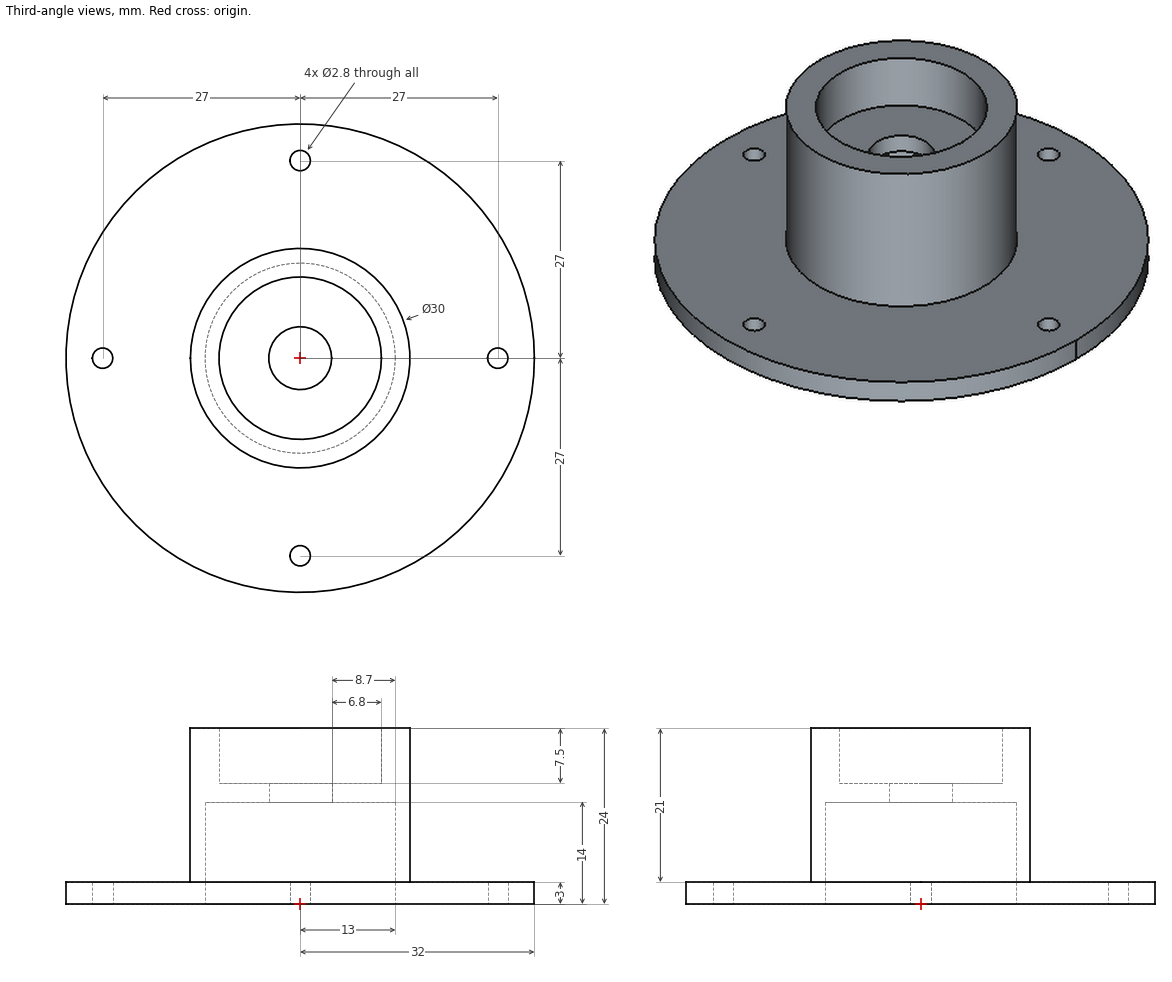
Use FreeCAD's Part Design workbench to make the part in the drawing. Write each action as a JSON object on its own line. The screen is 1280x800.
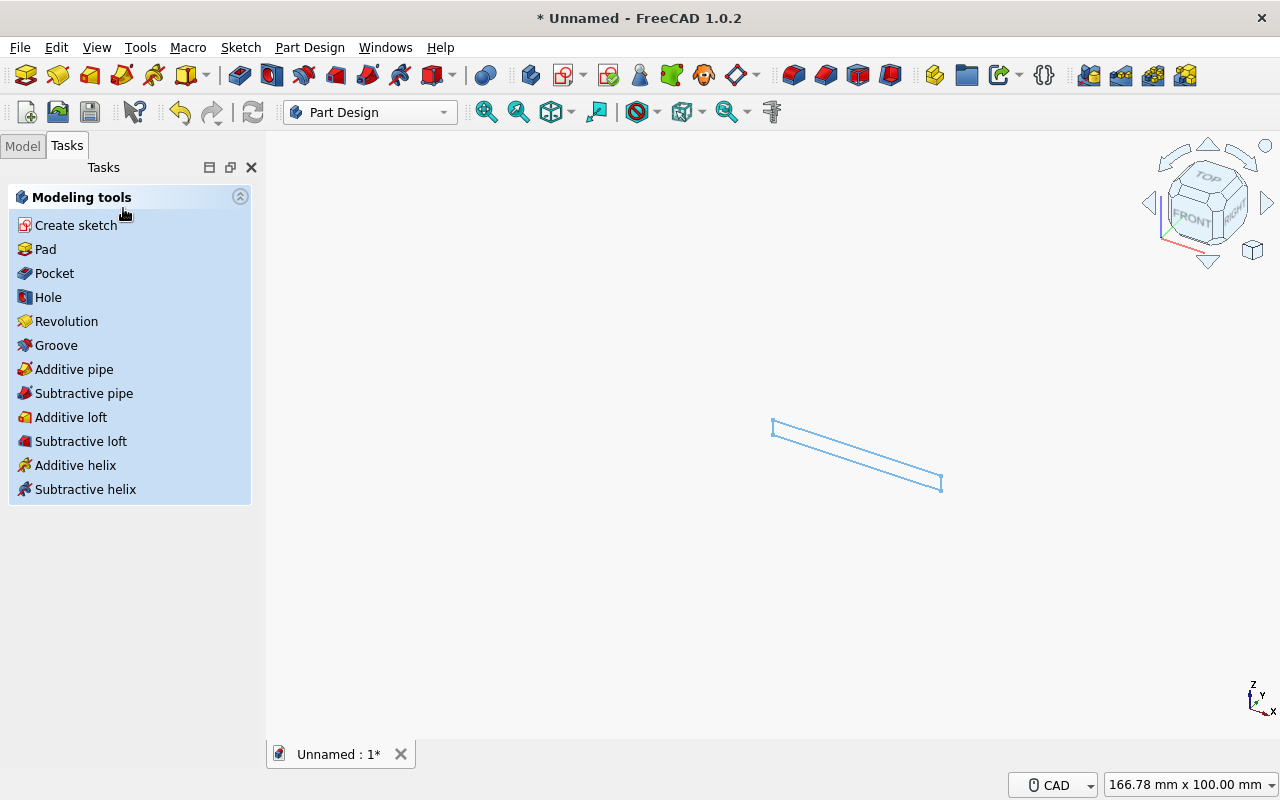
{"action": "left_click", "coordinate": [58, 76]}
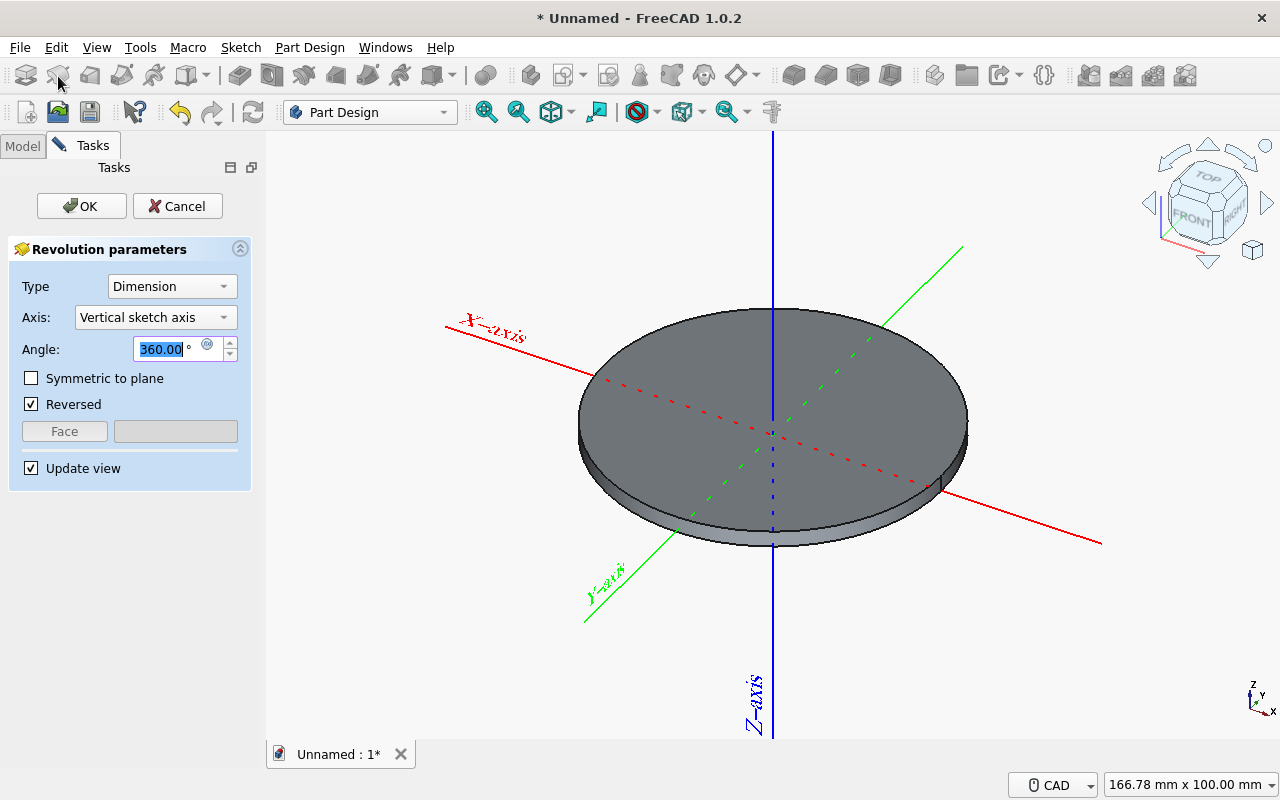
{"action": "left_click", "coordinate": [82, 206]}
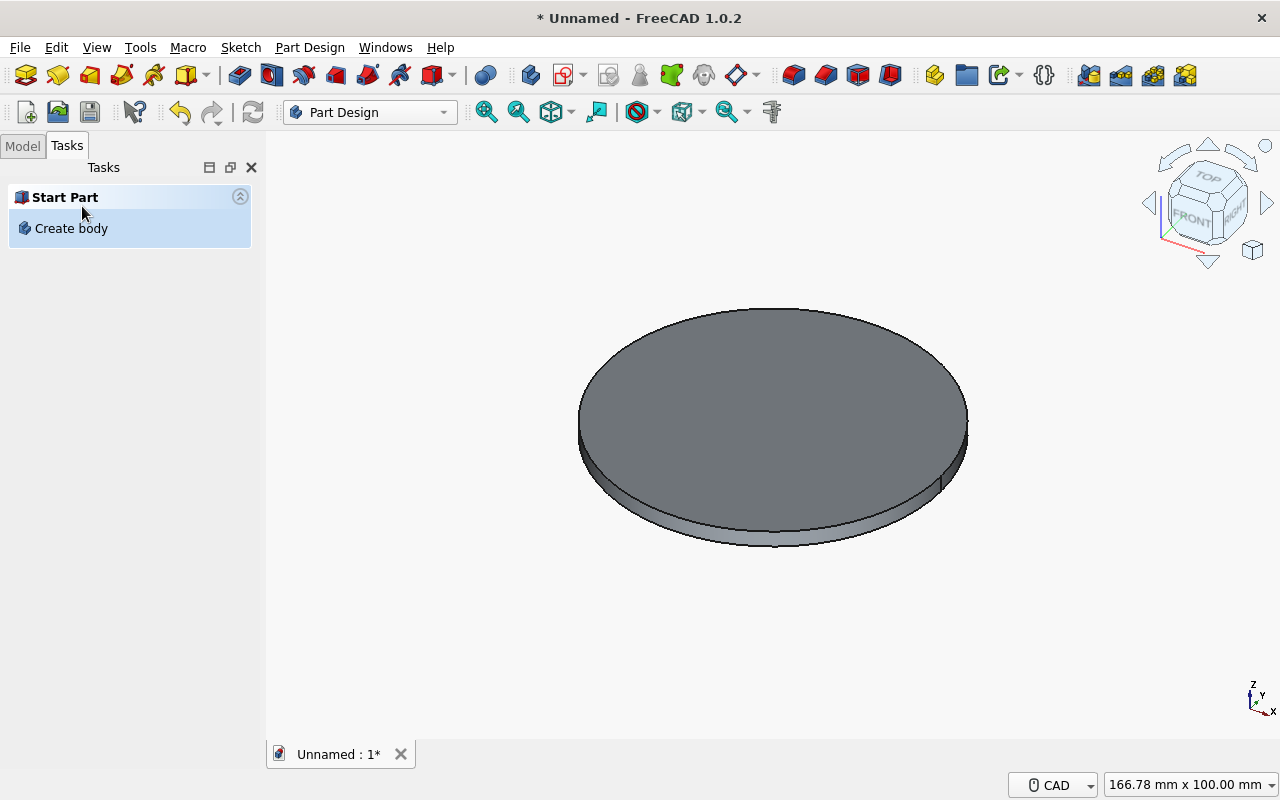
{"action": "left_click", "coordinate": [773, 419]}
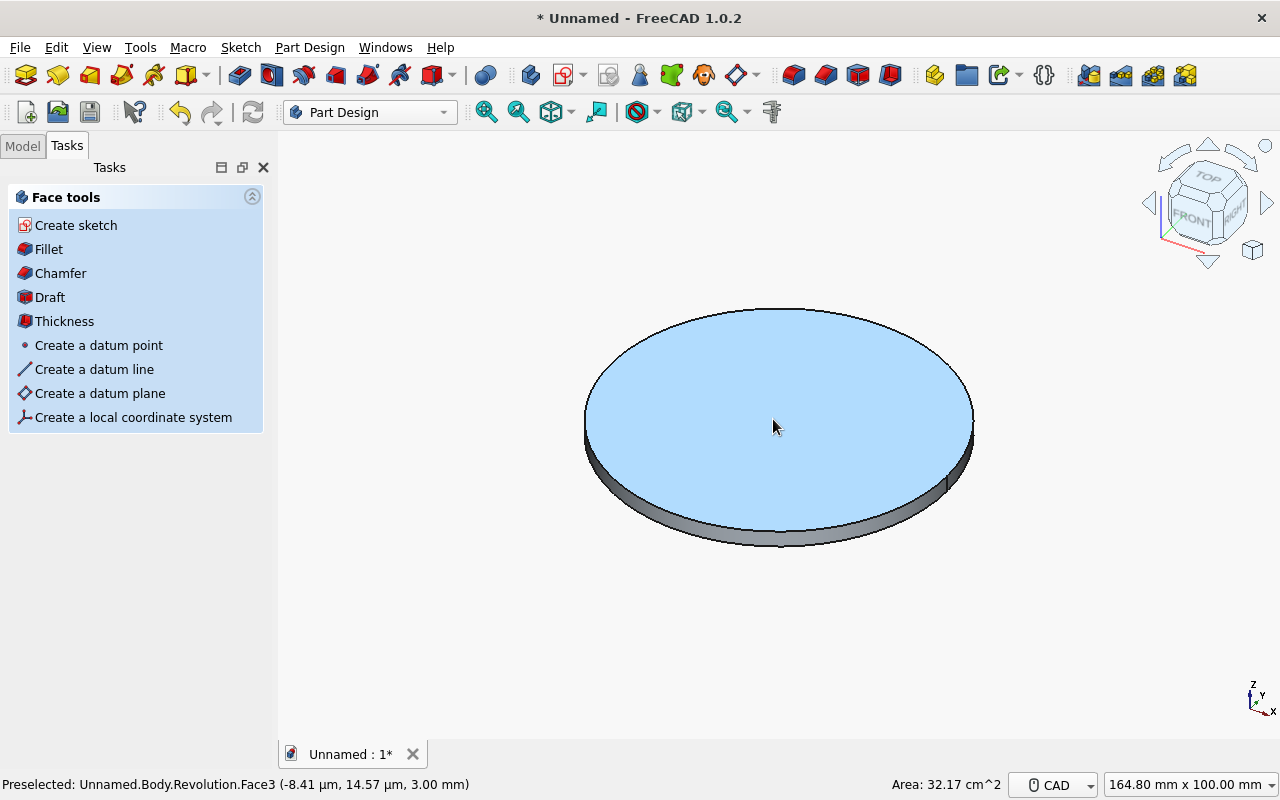
{"action": "left_click", "coordinate": [564, 76]}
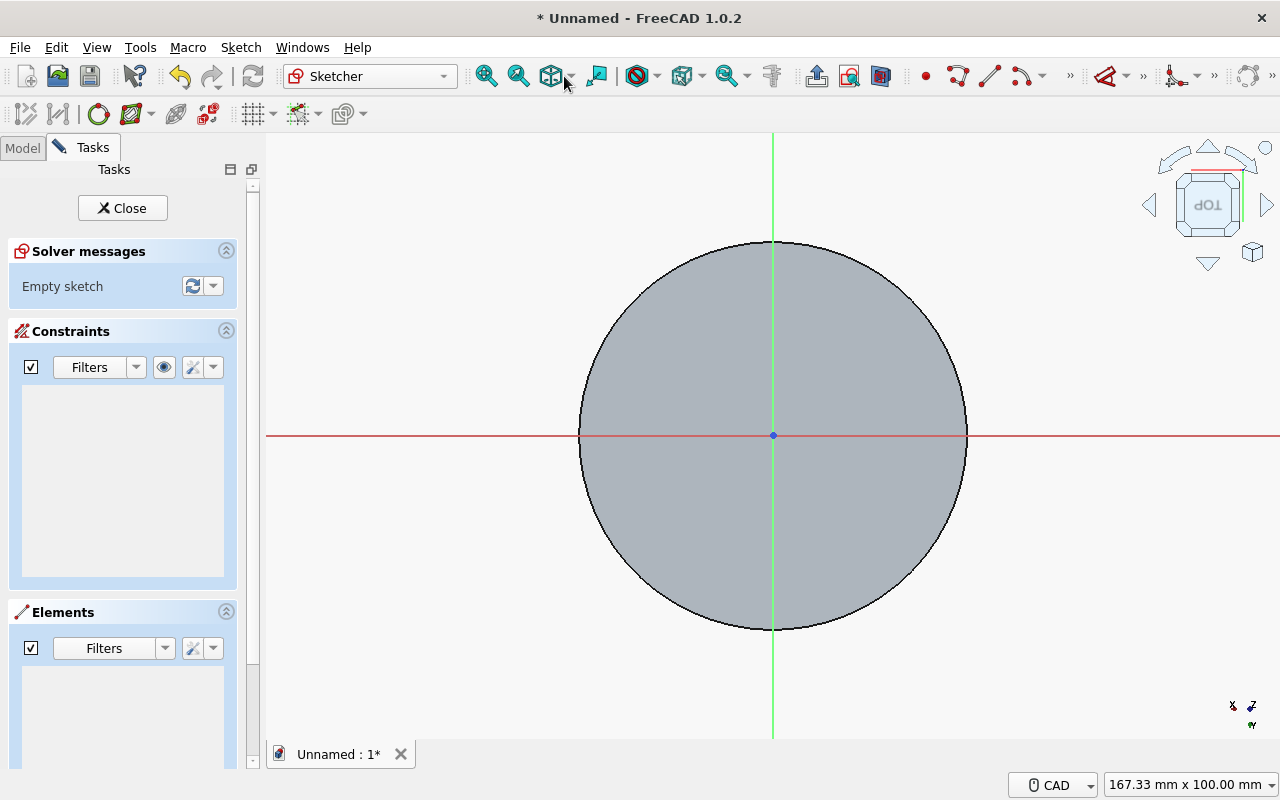
{"action": "scroll", "coordinate": [829, 436], "scroll_direction": "up", "scroll_amount": 4}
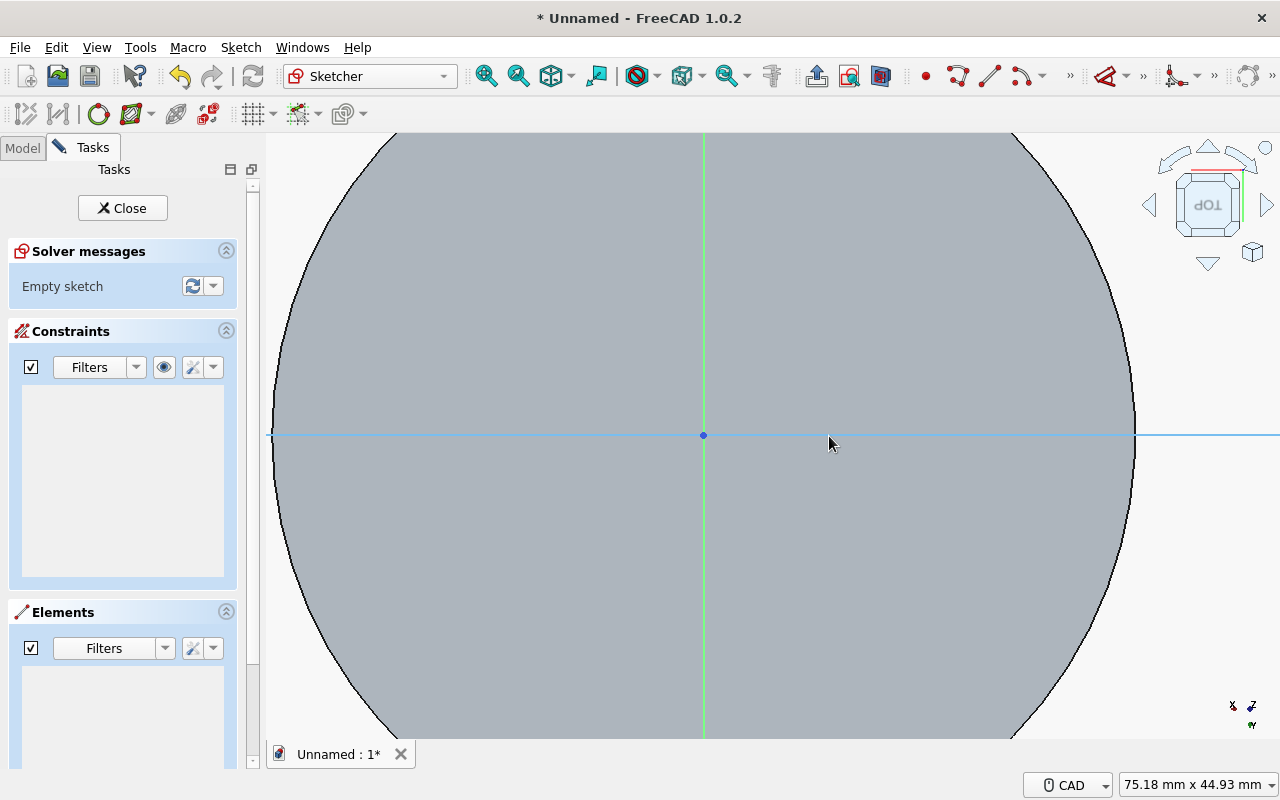
{"action": "key", "text": "g c"}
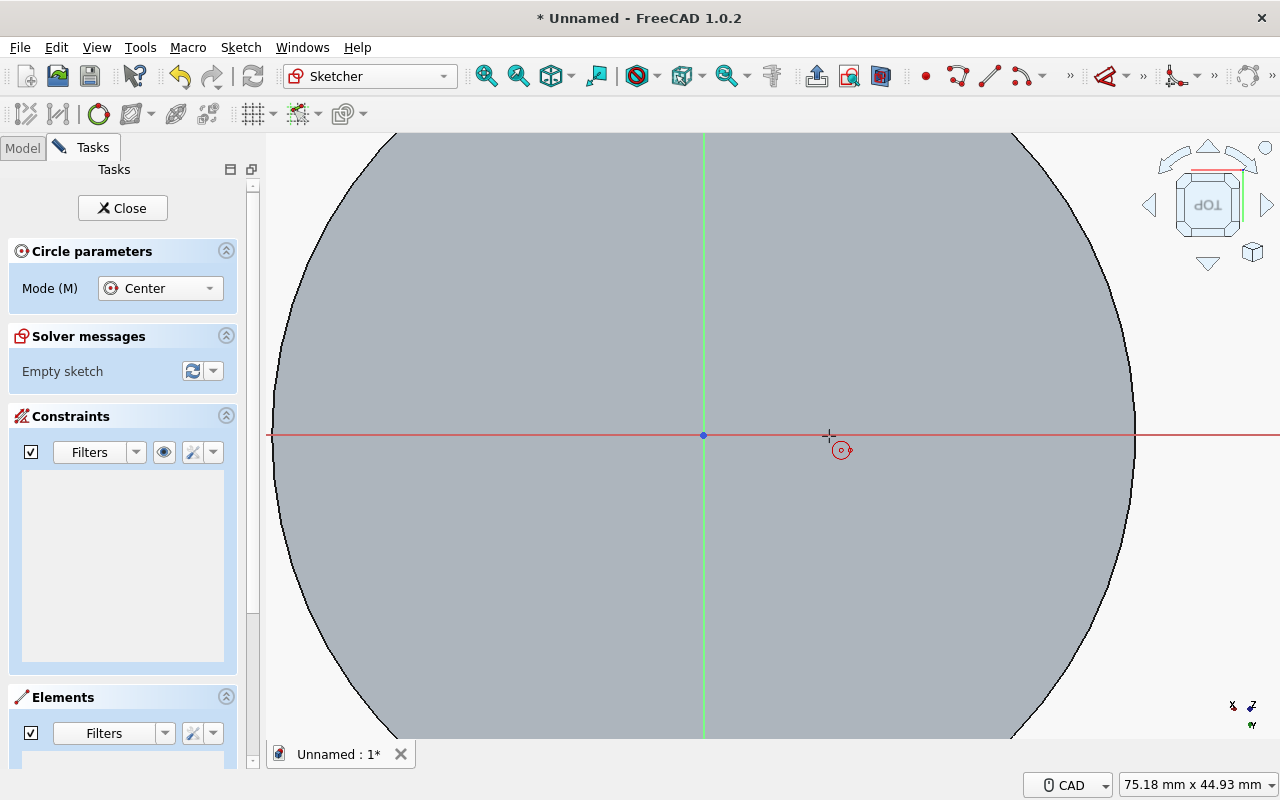
{"action": "left_click", "coordinate": [704, 435]}
{"action": "mouse_move", "coordinate": [847, 292]}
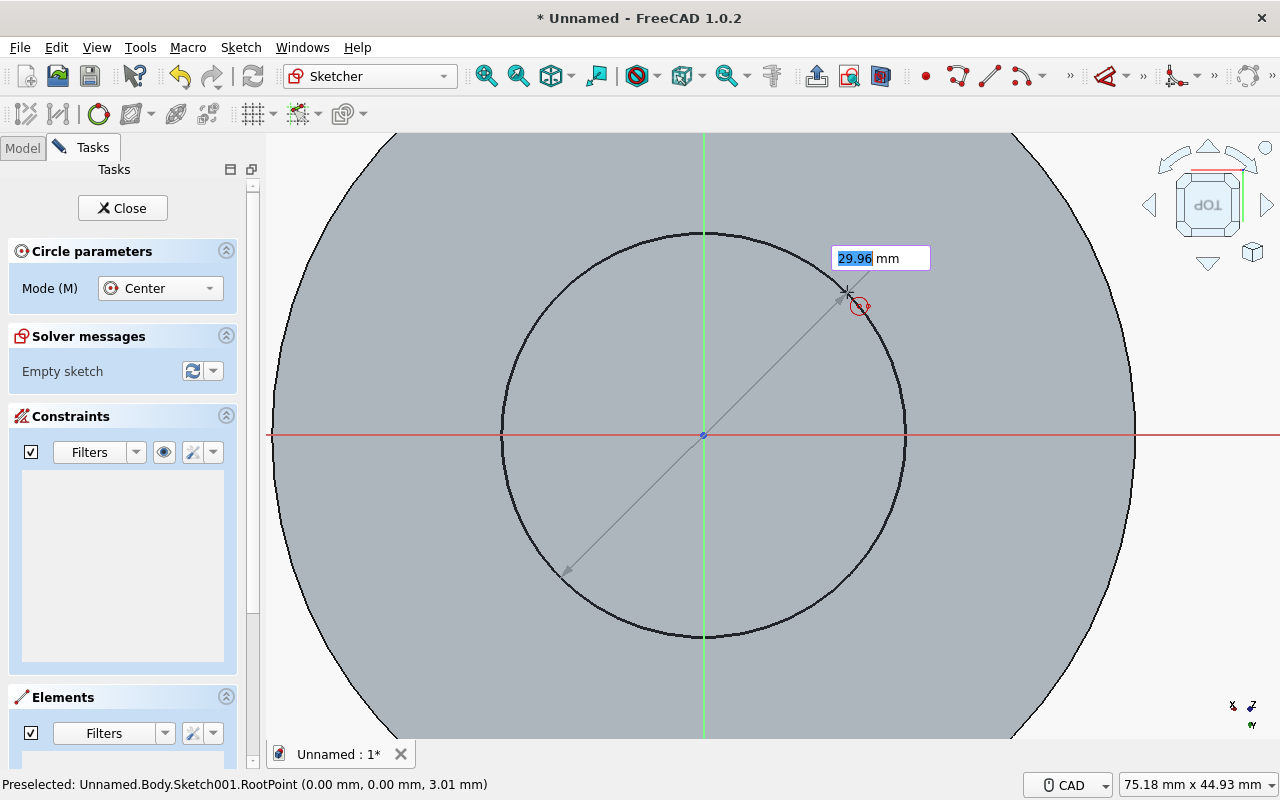
{"action": "type", "text": "30"}
{"action": "key", "text": "Return"}
{"action": "key", "text": "Escape"}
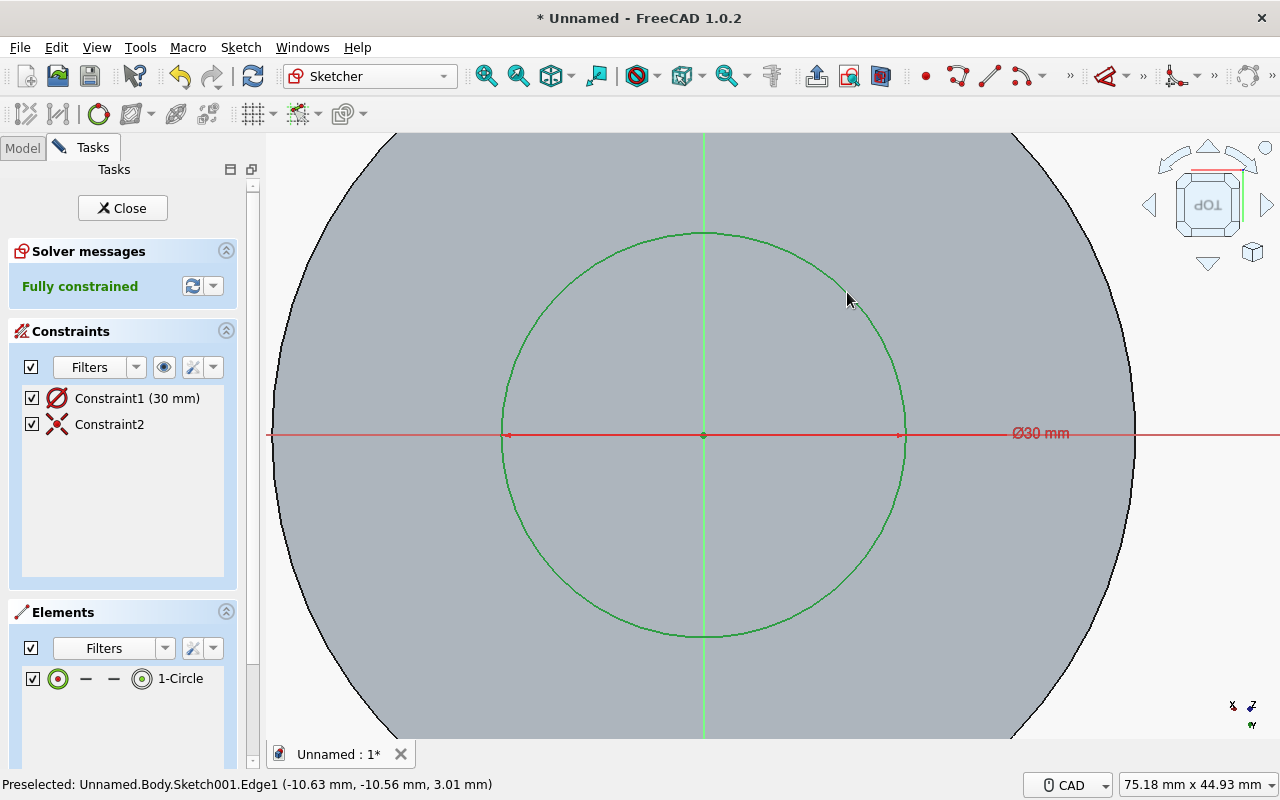
{"action": "left_click", "coordinate": [123, 208]}